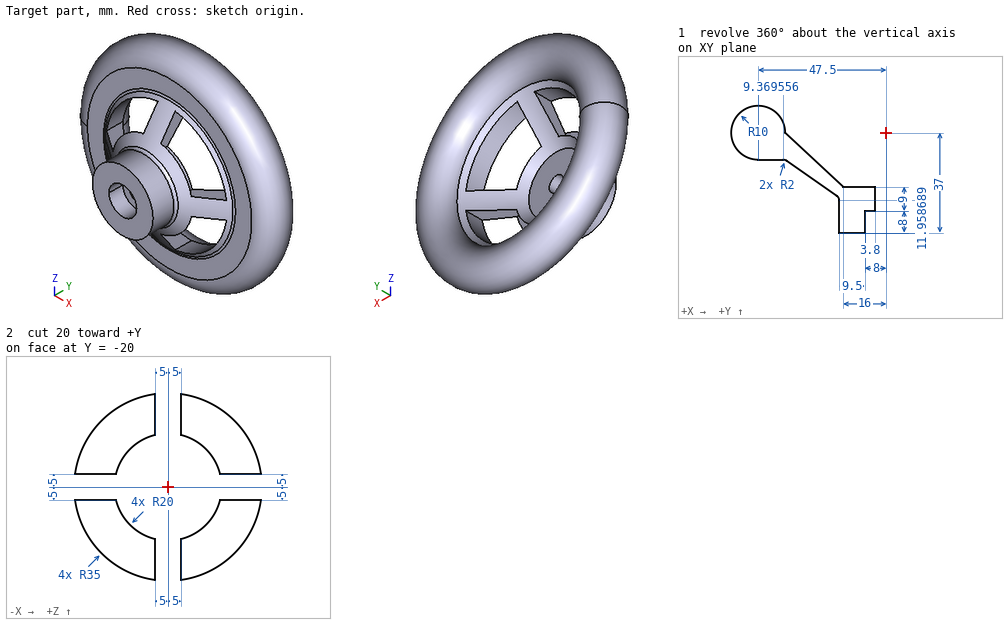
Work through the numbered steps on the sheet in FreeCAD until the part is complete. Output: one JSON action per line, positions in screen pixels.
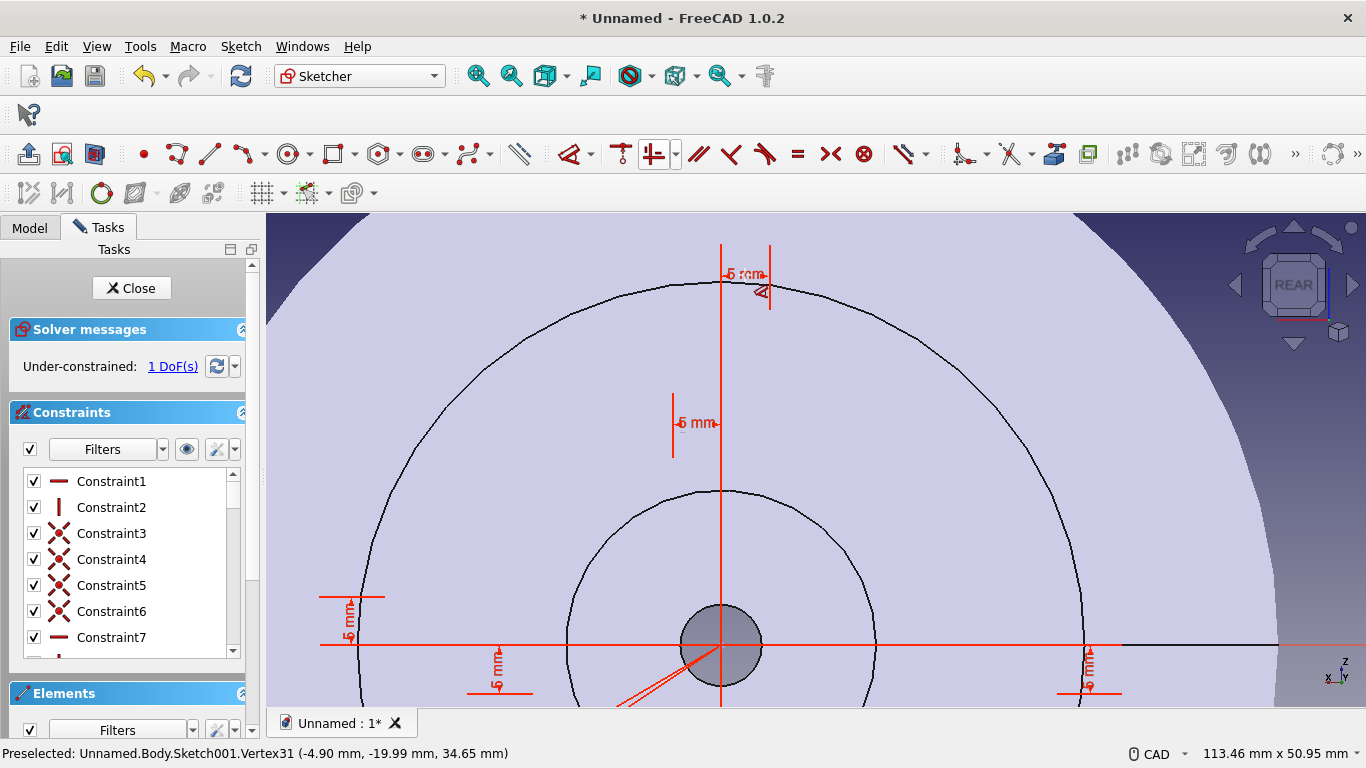
{"action": "left_click", "coordinate": [910, 600]}
{"action": "left_click", "coordinate": [944, 623]}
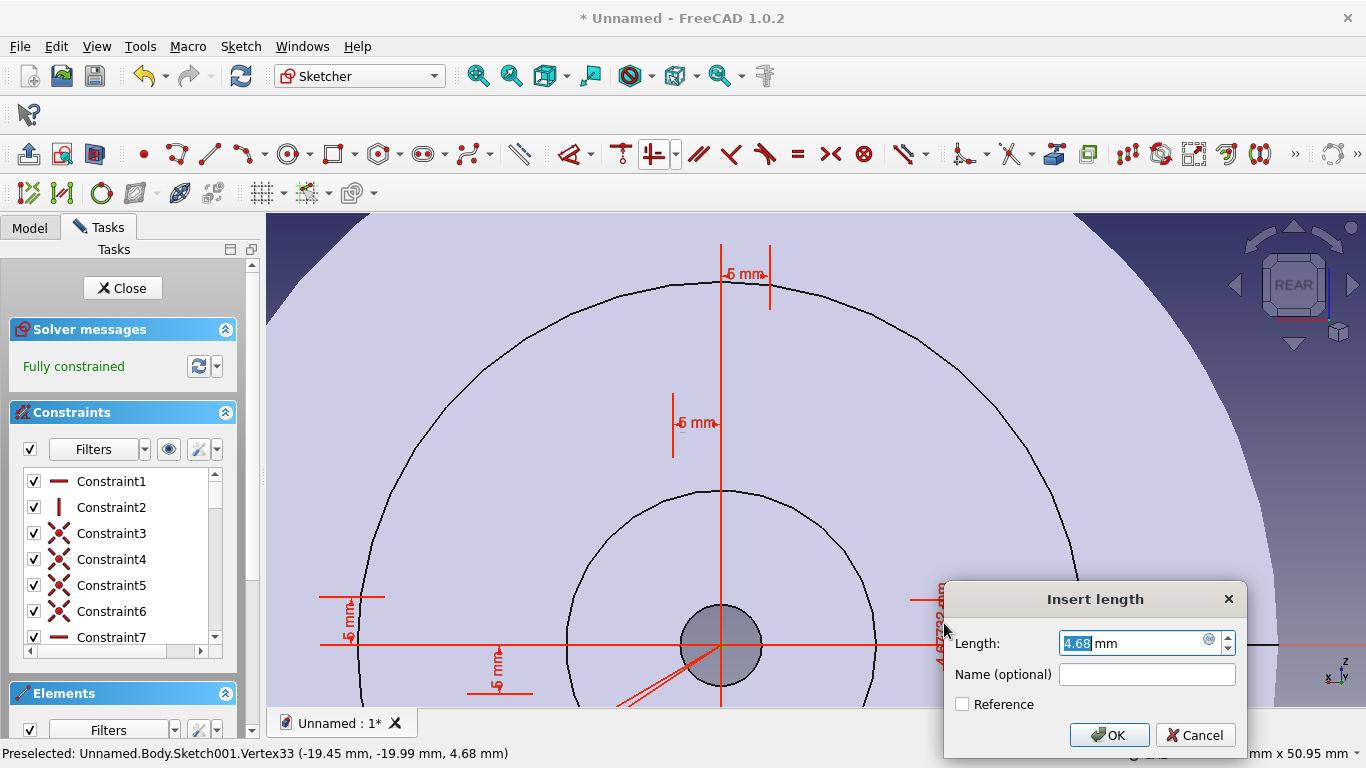
{"action": "type", "text": "5"}
{"action": "key", "text": "Return"}
{"action": "key", "text": "Escape"}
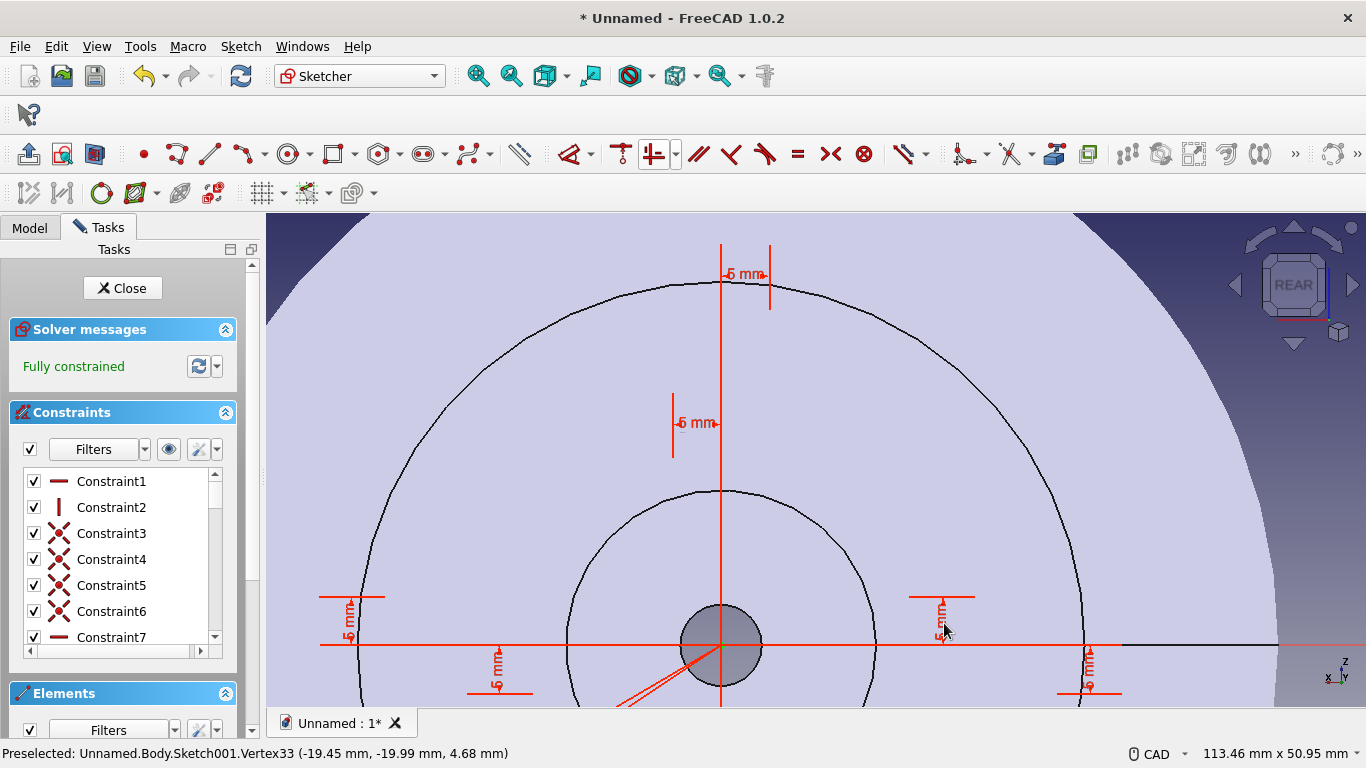
{"action": "left_click", "coordinate": [123, 288]}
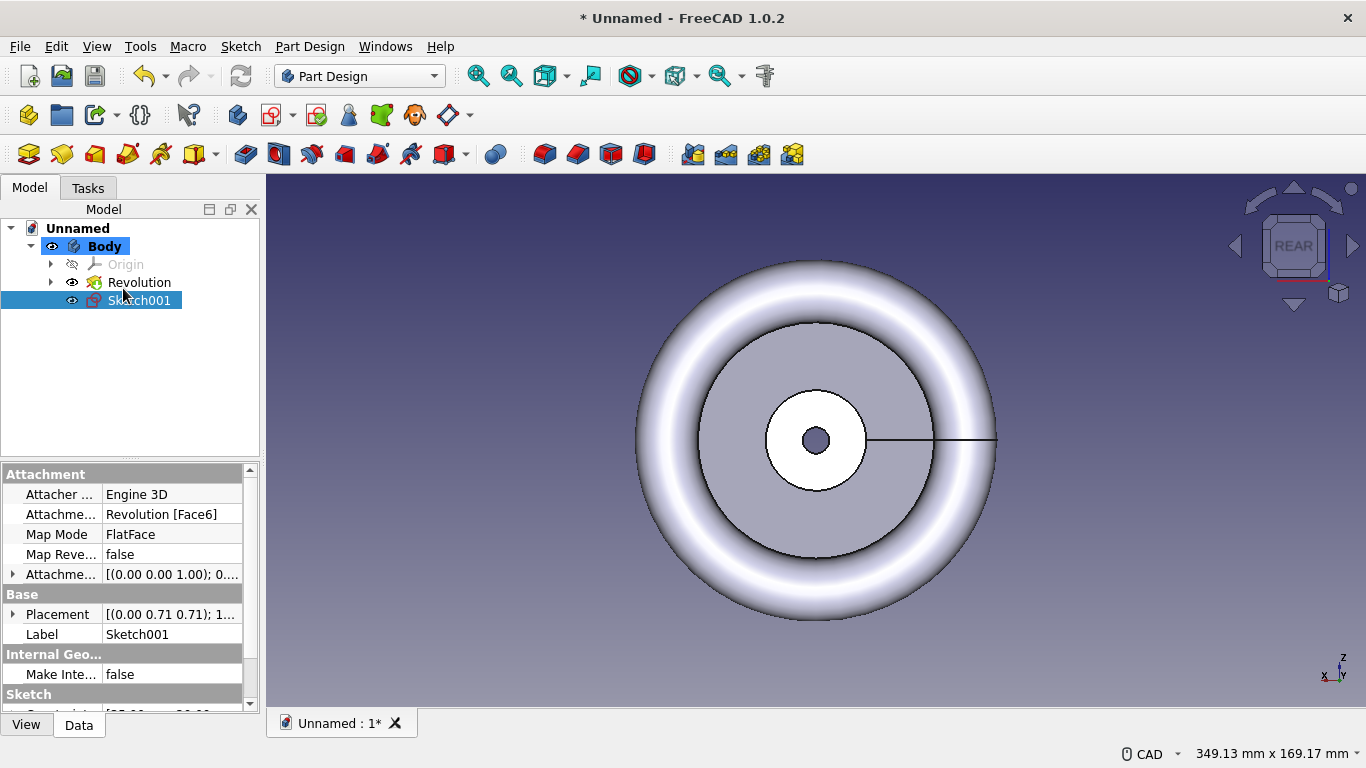
{"action": "left_click", "coordinate": [246, 154]}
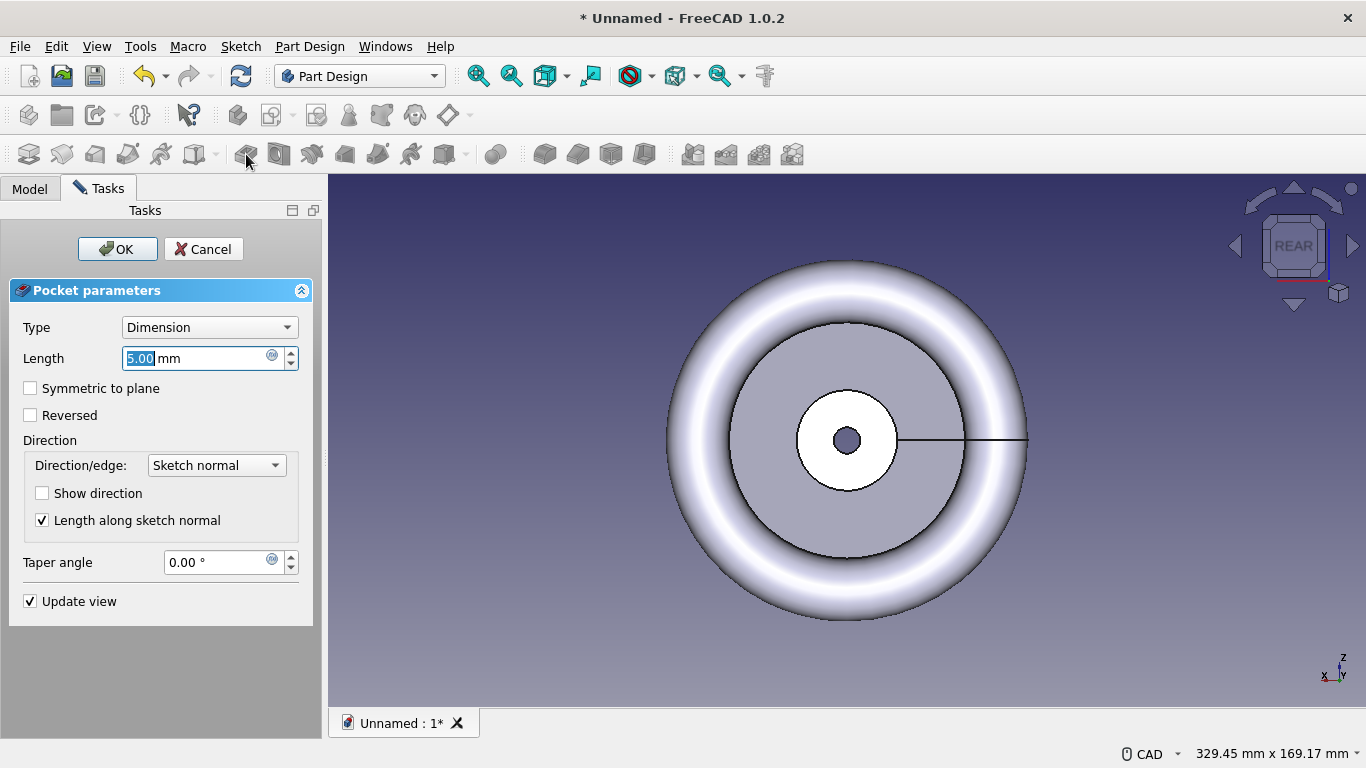
{"action": "type", "text": "20"}
{"action": "key", "text": "Tab"}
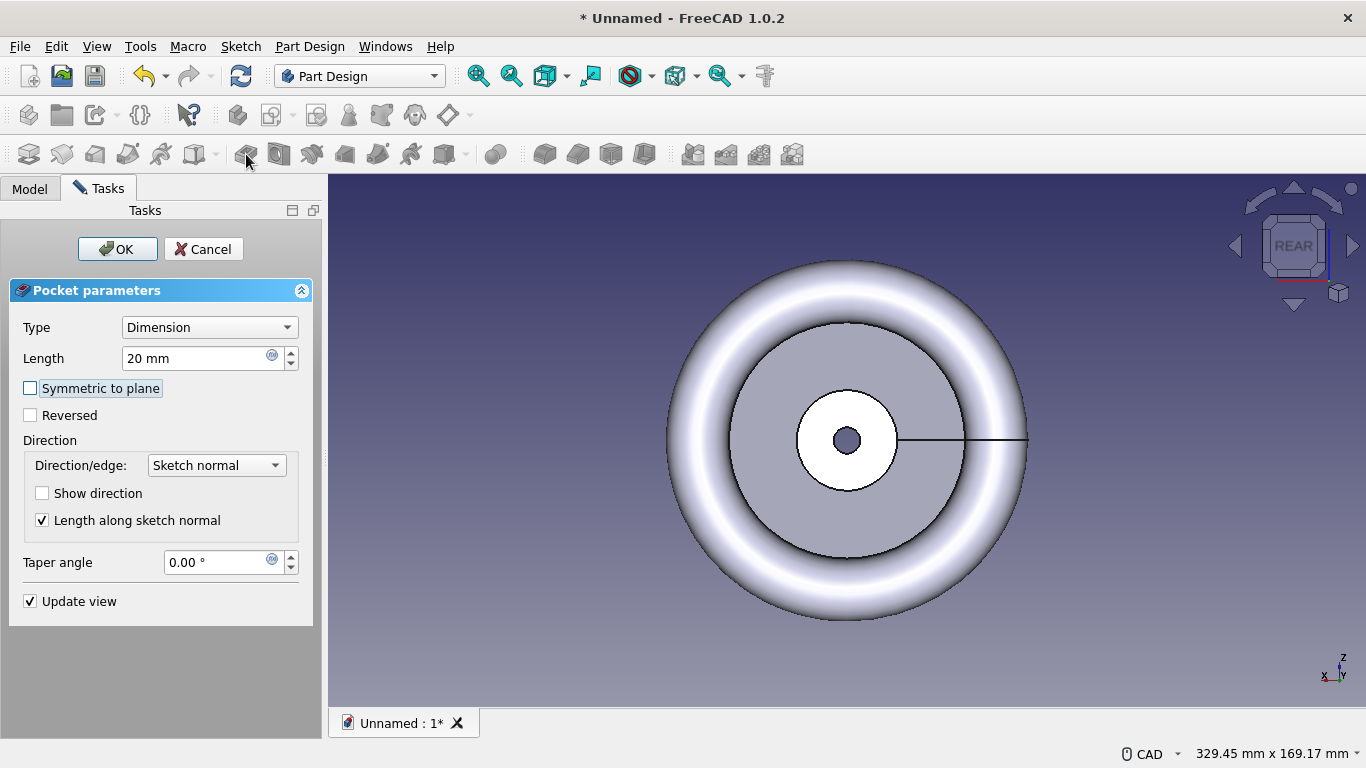
{"action": "left_click", "coordinate": [31, 415]}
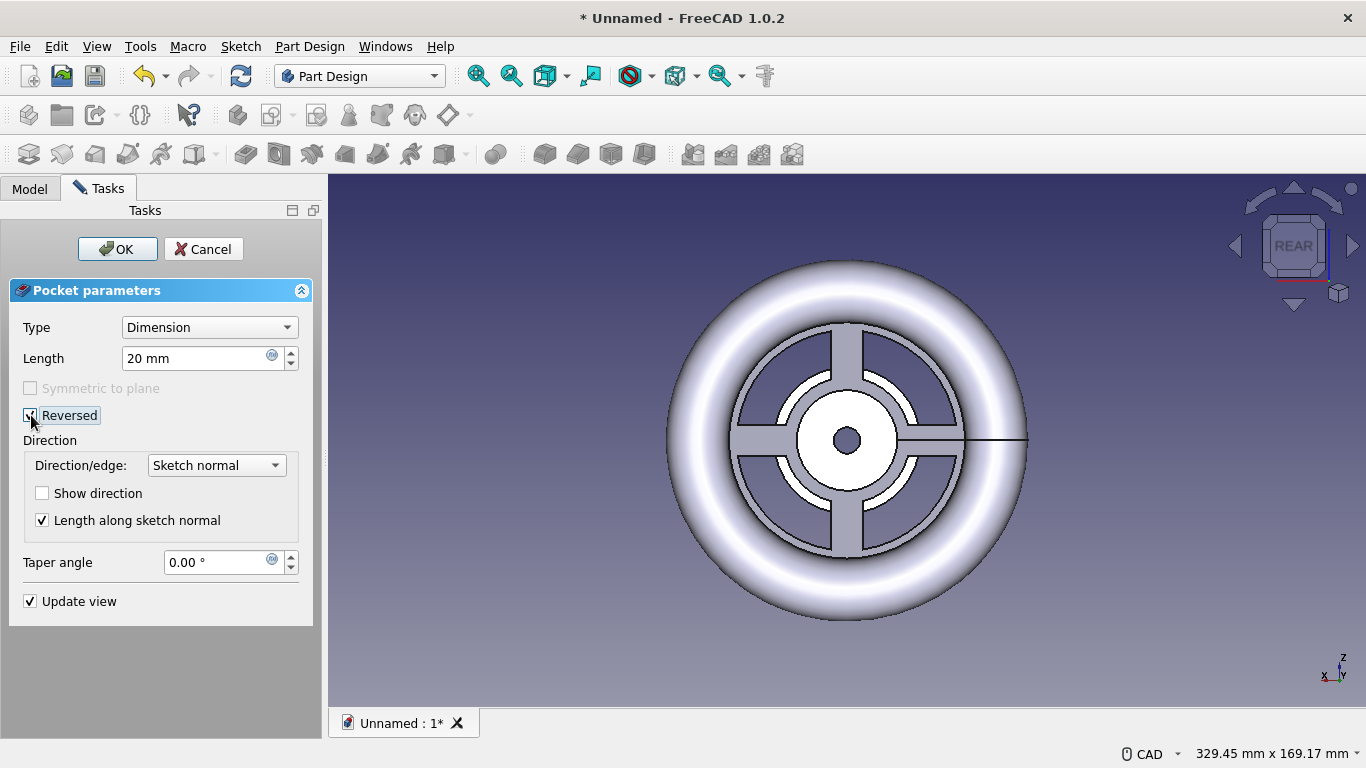
{"action": "left_click", "coordinate": [118, 249]}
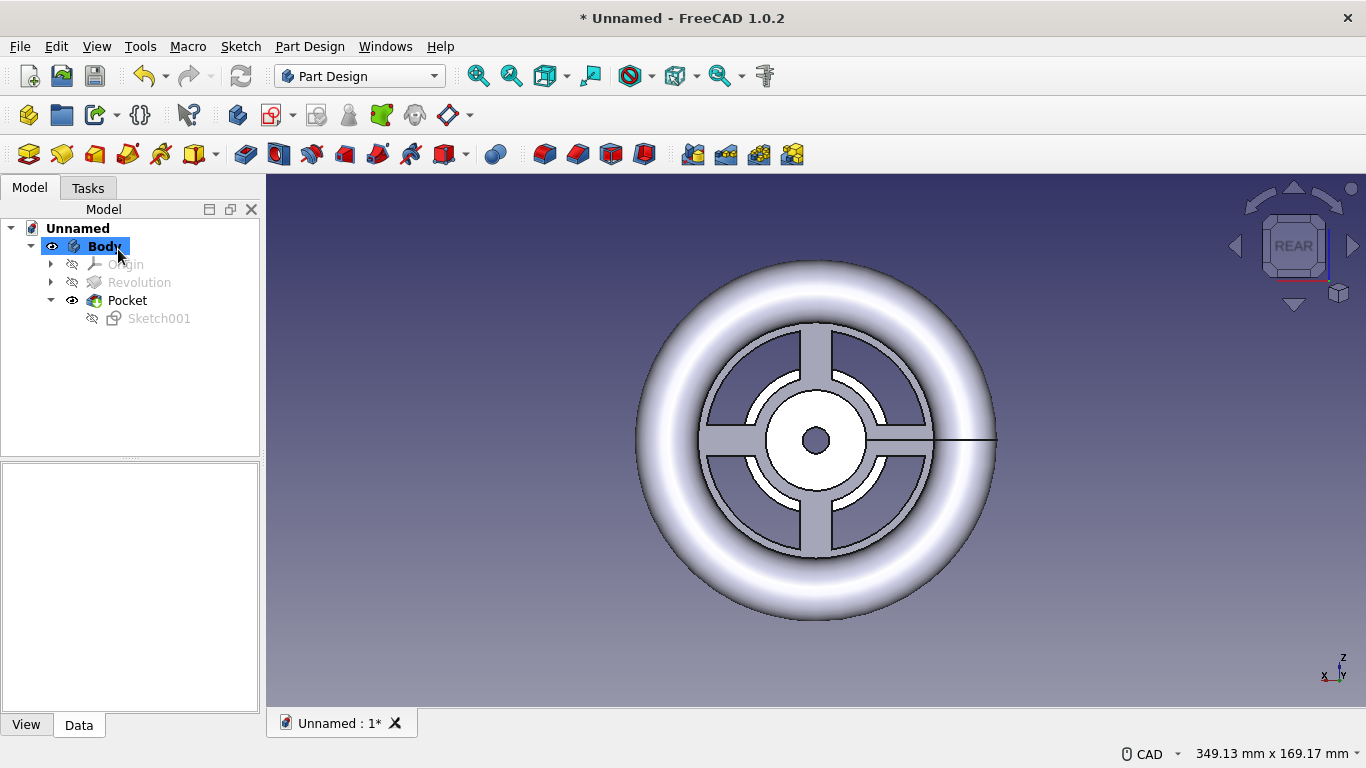
{"action": "key", "text": "0"}